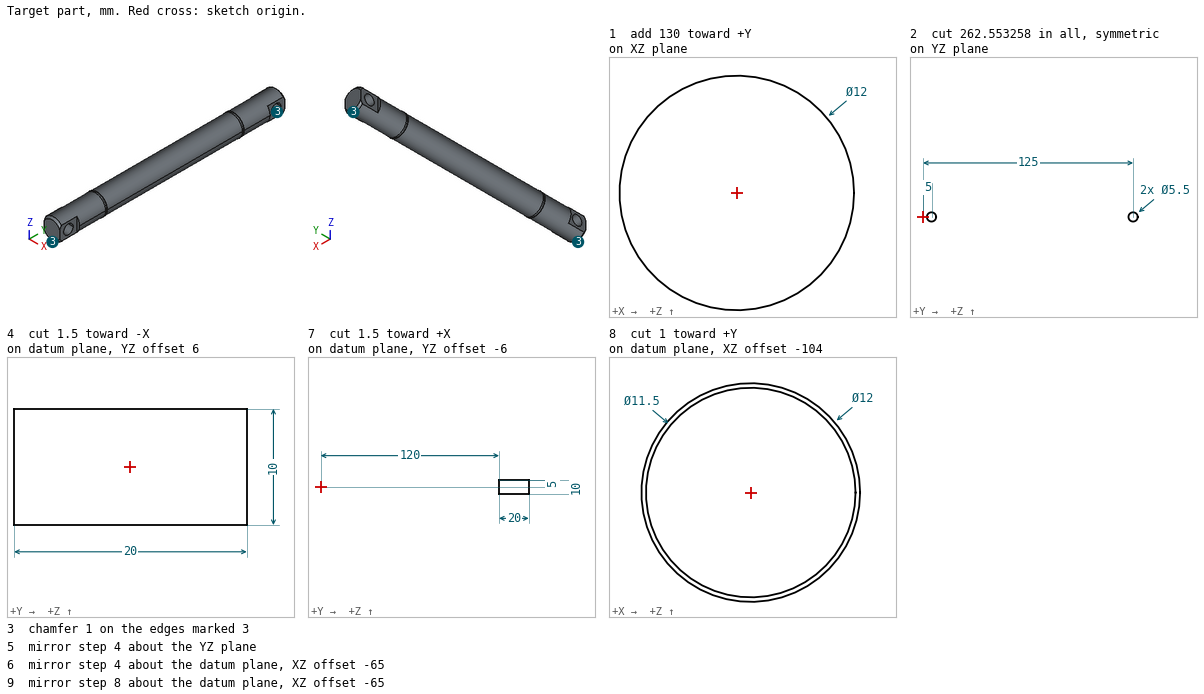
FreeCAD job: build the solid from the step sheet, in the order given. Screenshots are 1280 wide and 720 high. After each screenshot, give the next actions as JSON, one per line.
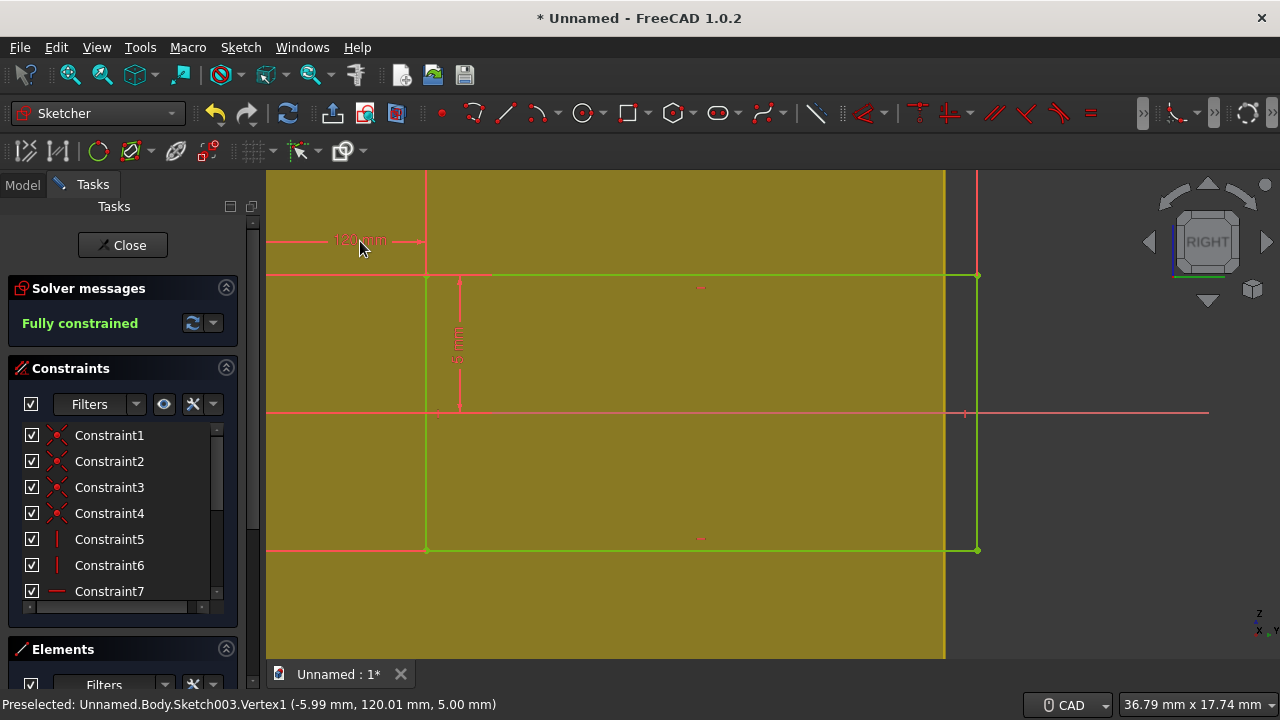
{"action": "left_click", "coordinate": [123, 245]}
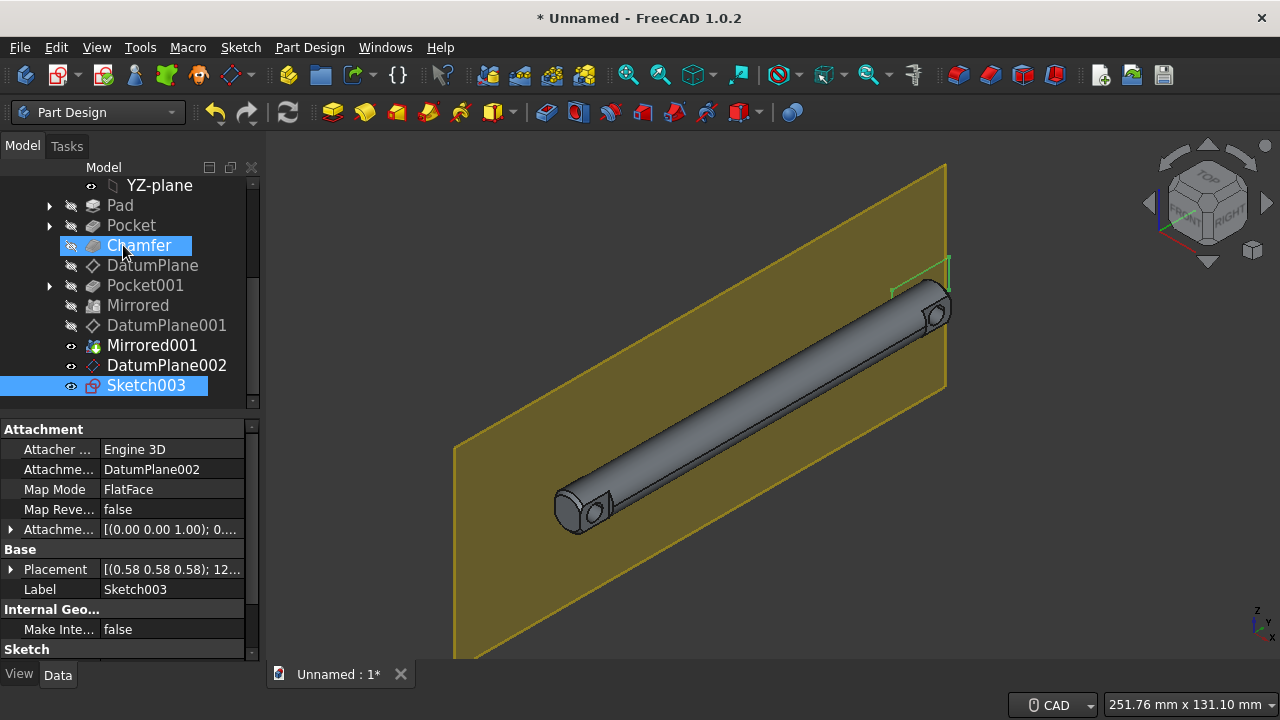
{"action": "left_click", "coordinate": [548, 112]}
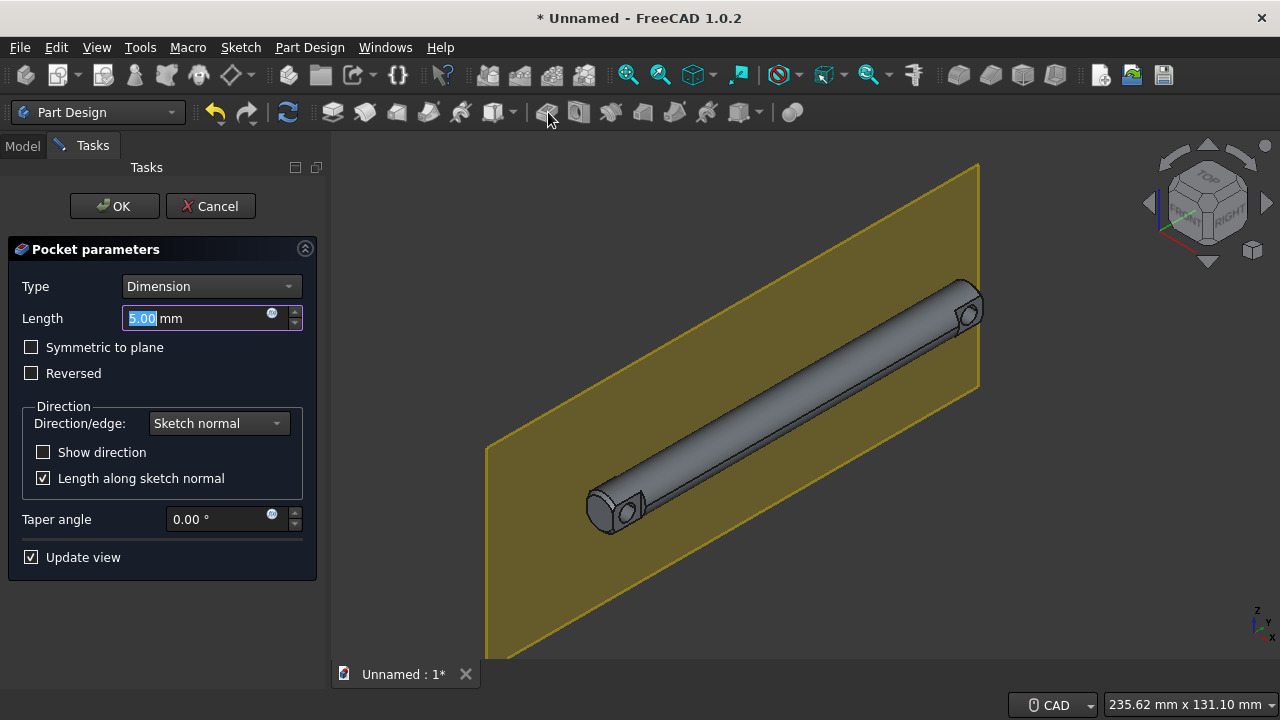
{"action": "type", "text": "1.5"}
{"action": "key", "text": "Tab"}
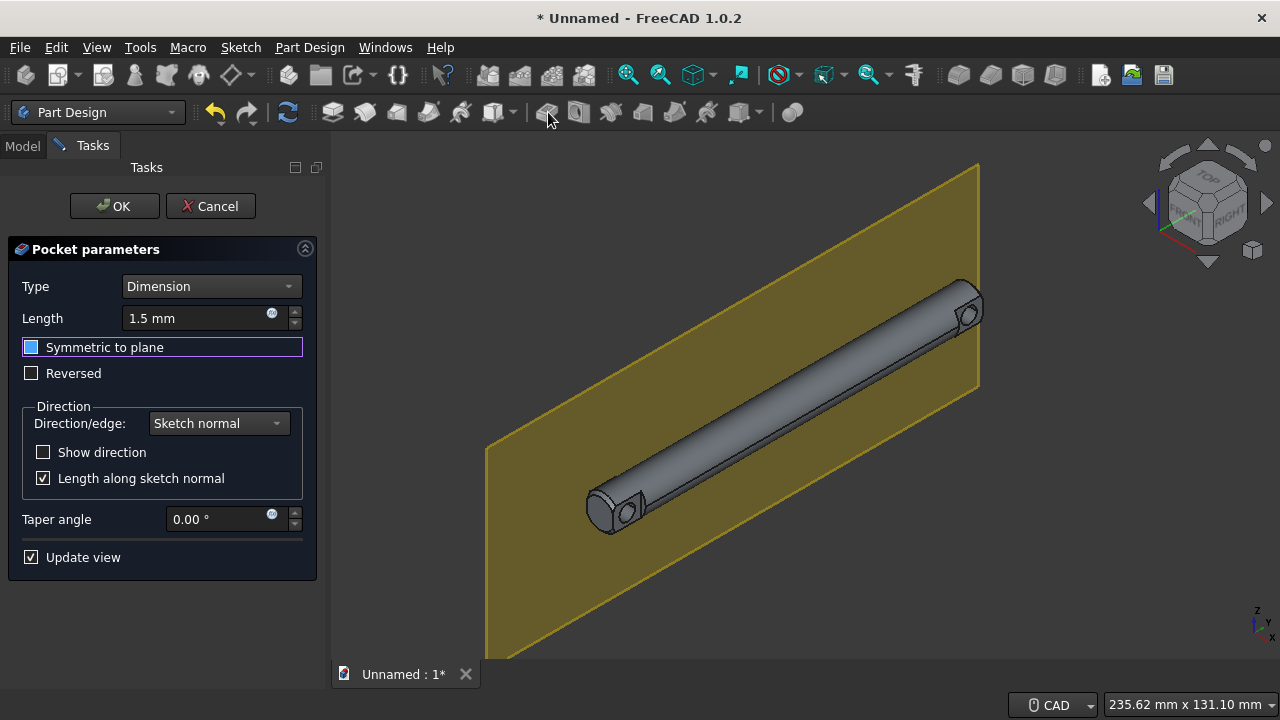
{"action": "left_click", "coordinate": [30, 373]}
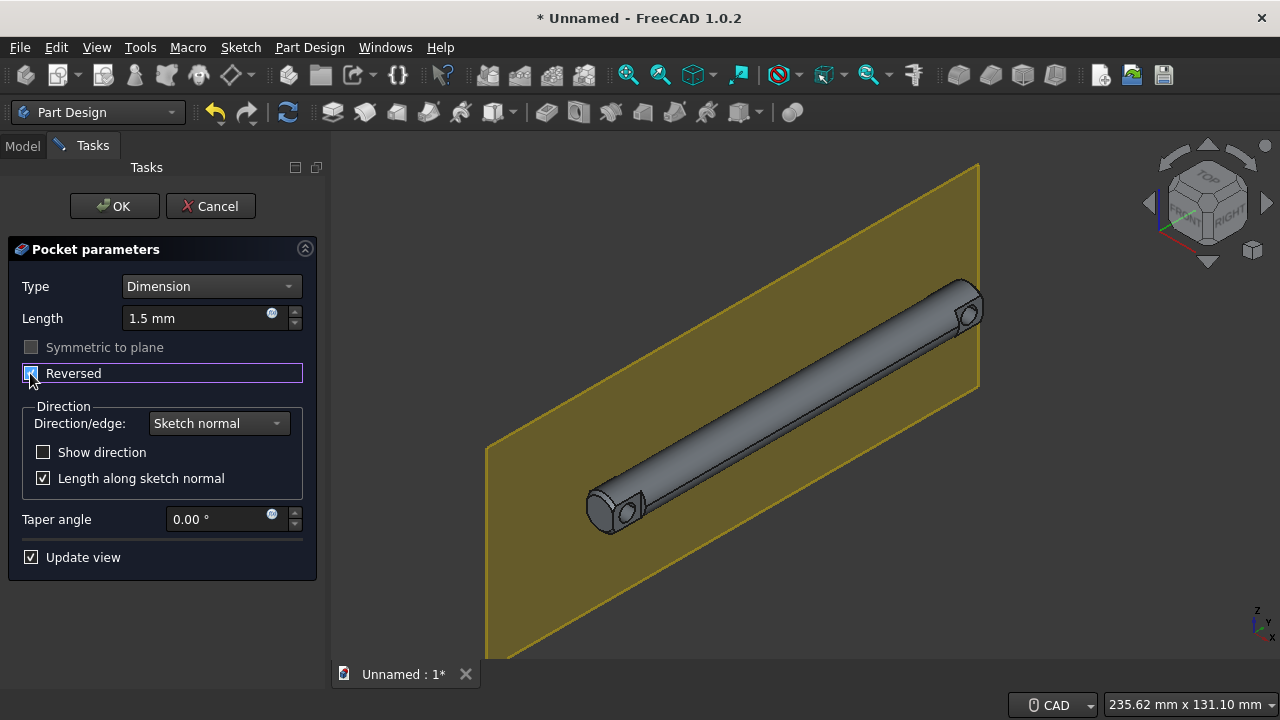
{"action": "left_click", "coordinate": [115, 206]}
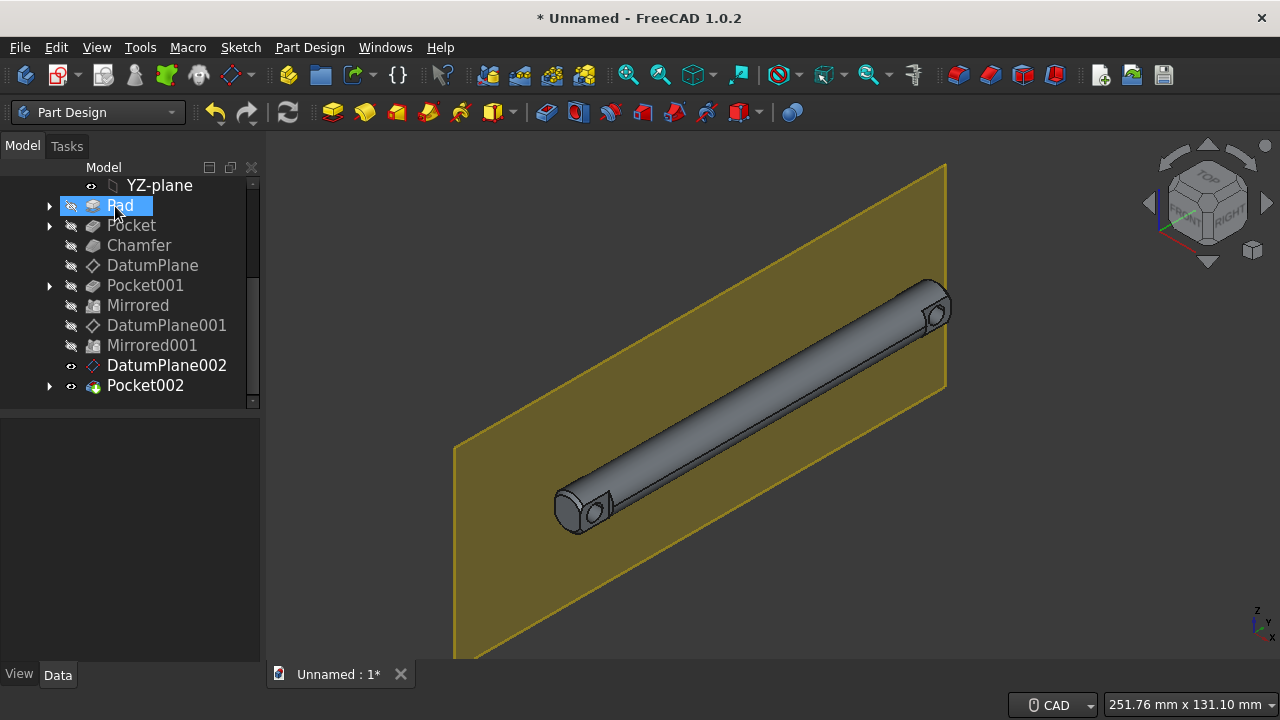
{"action": "left_click", "coordinate": [116, 366]}
{"action": "key", "text": "space"}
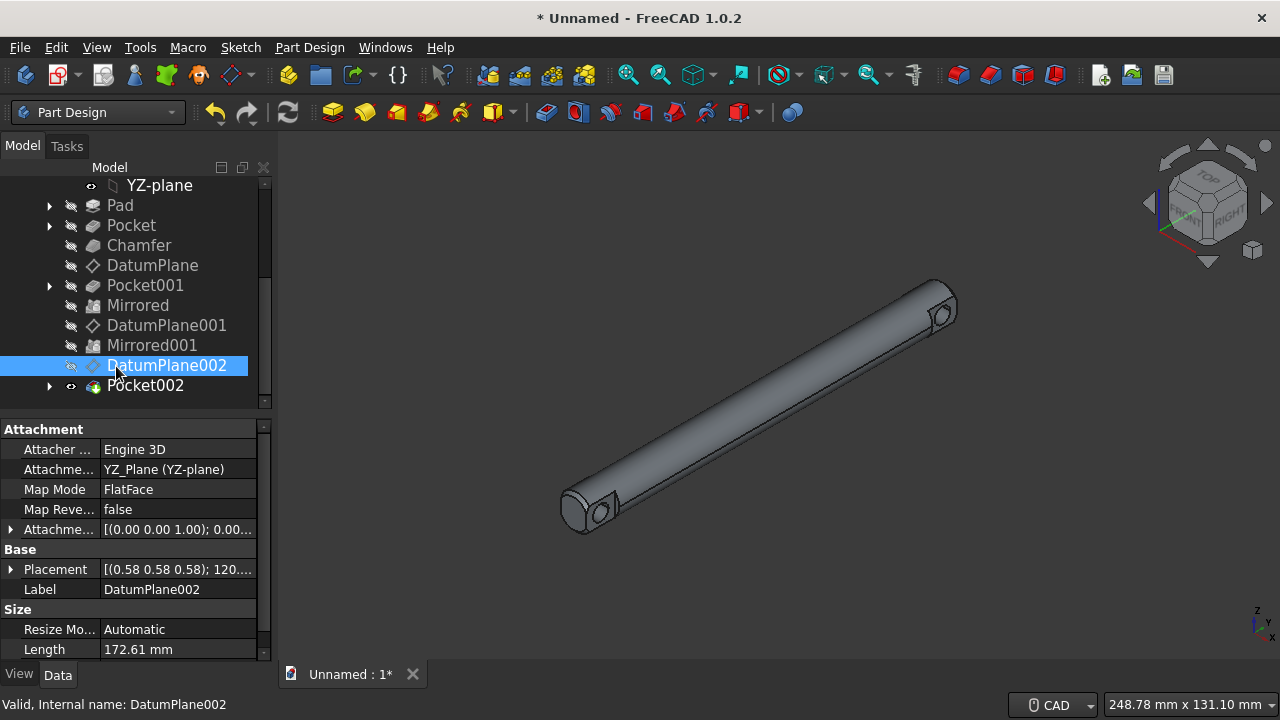
{"action": "scroll", "coordinate": [160, 281], "scroll_direction": "down", "scroll_amount": 3}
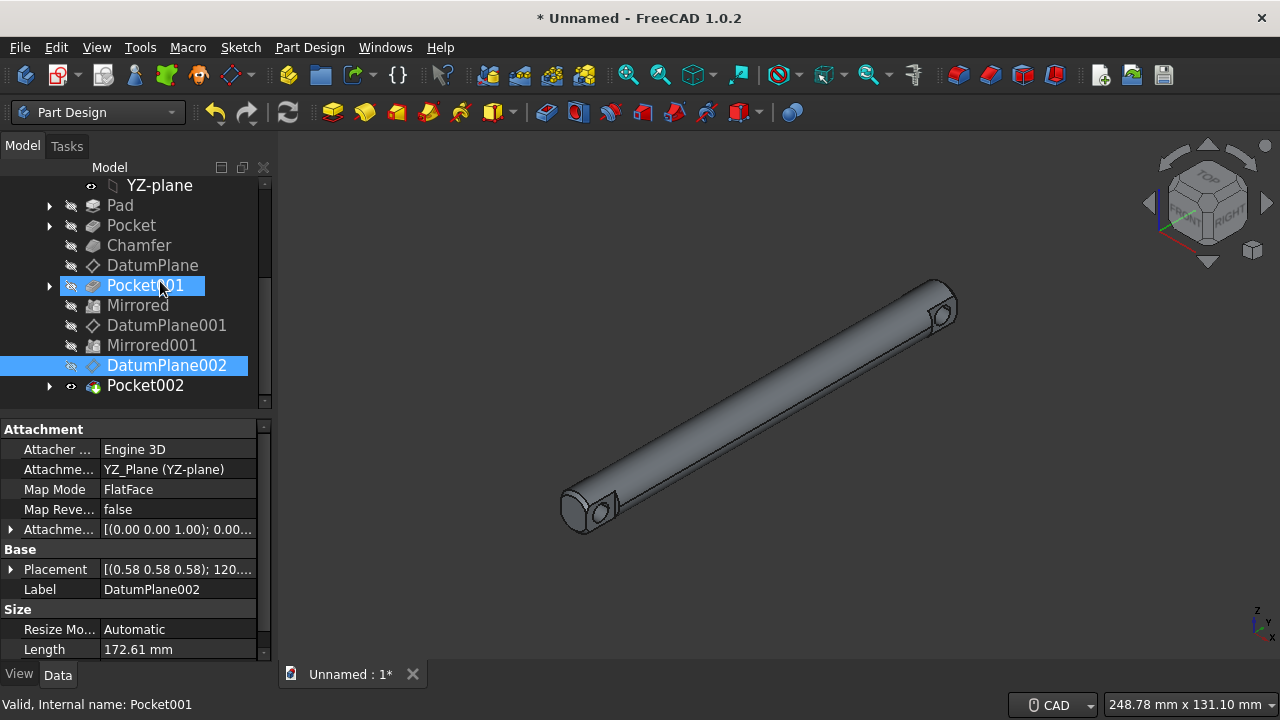
{"action": "scroll", "coordinate": [160, 281], "scroll_direction": "up", "scroll_amount": 15}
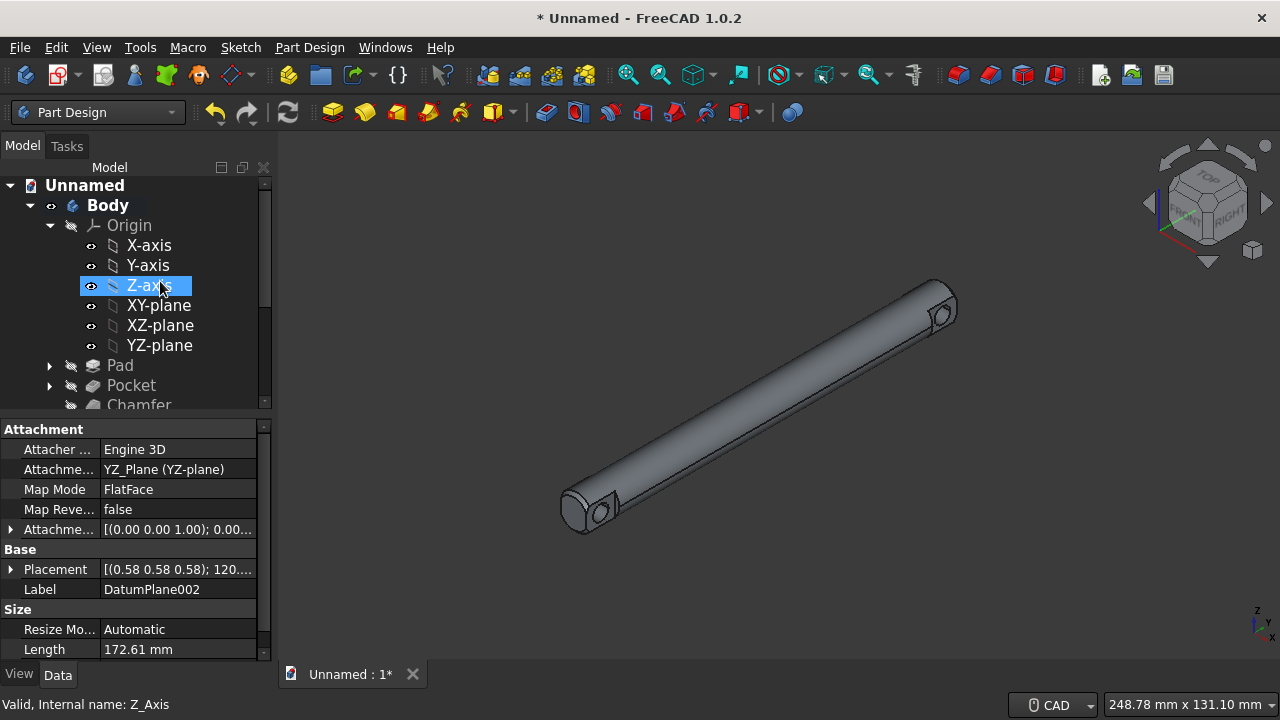
{"action": "left_click", "coordinate": [136, 326]}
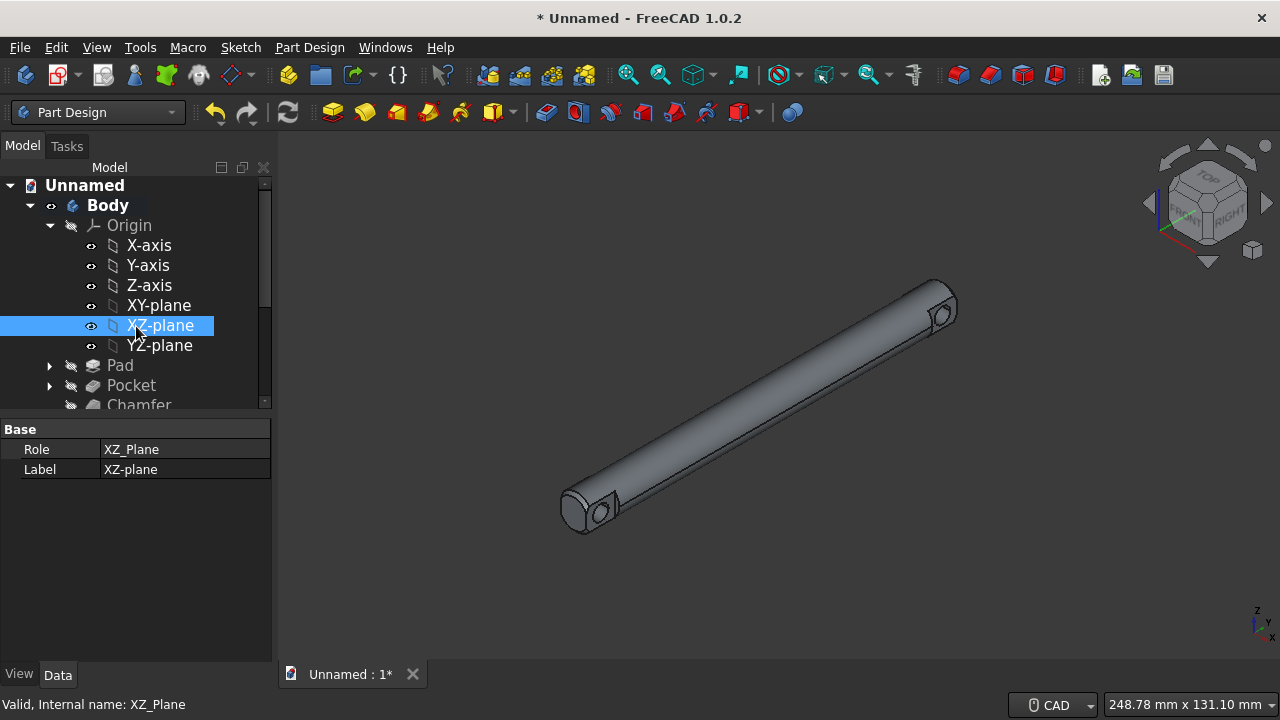
{"action": "left_click", "coordinate": [232, 76]}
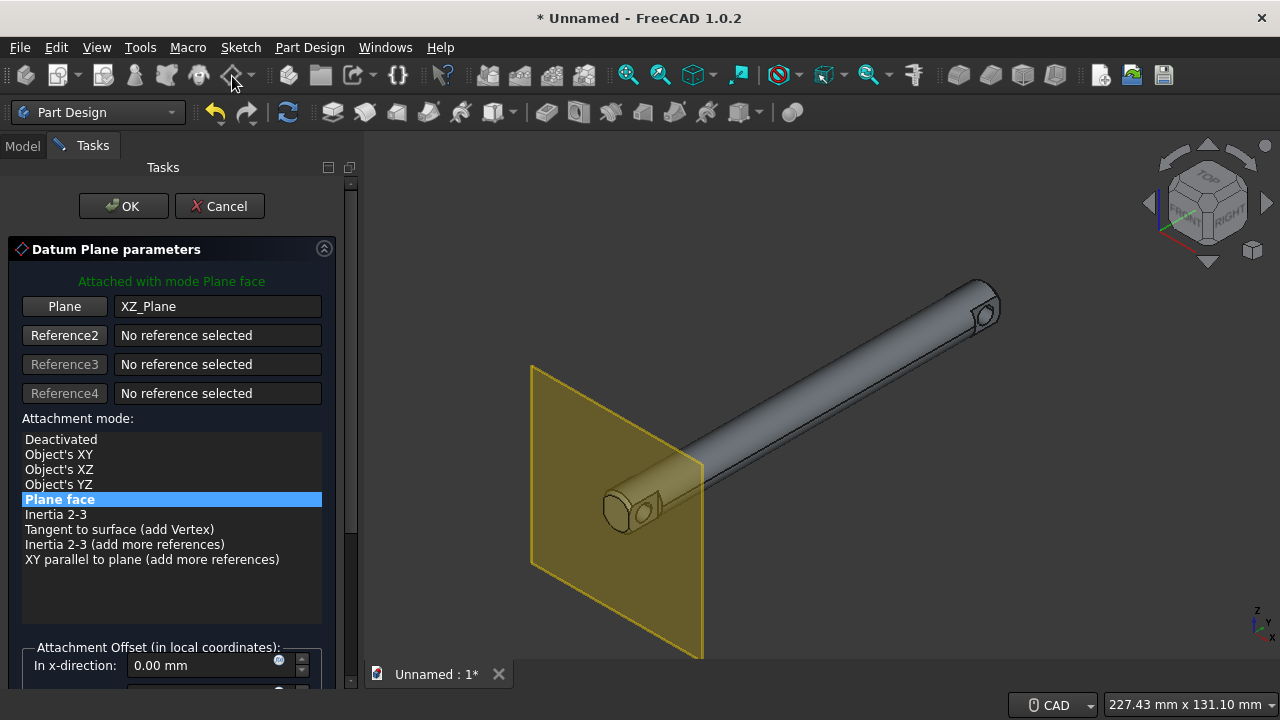
{"action": "scroll", "coordinate": [351, 432], "scroll_direction": "down", "scroll_amount": 2}